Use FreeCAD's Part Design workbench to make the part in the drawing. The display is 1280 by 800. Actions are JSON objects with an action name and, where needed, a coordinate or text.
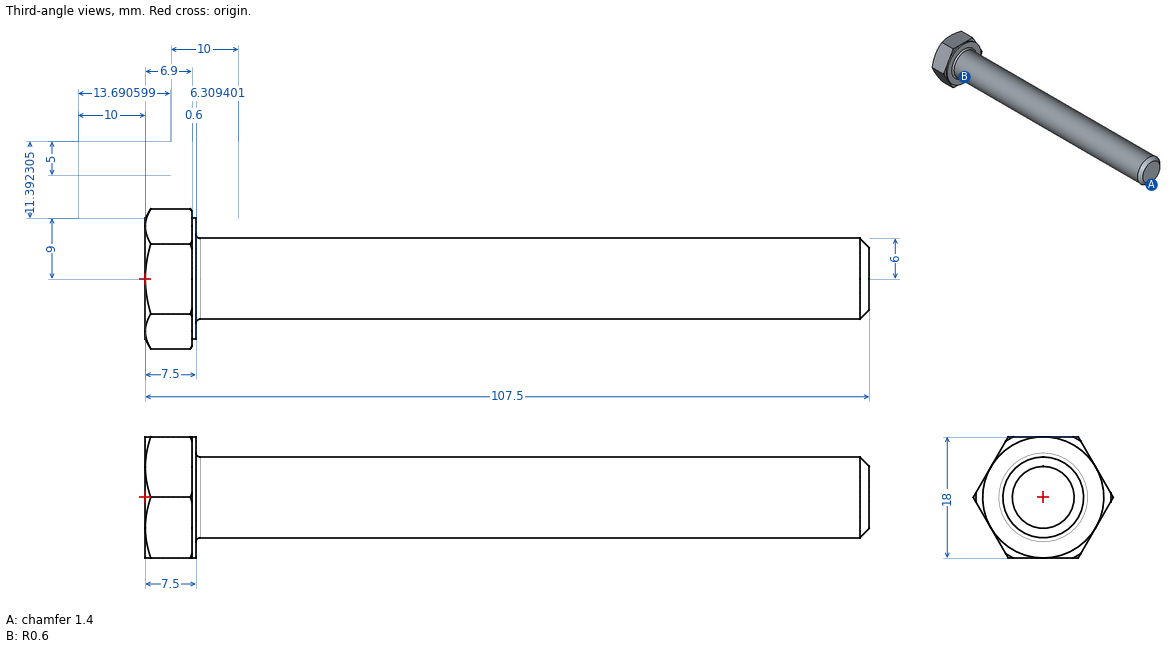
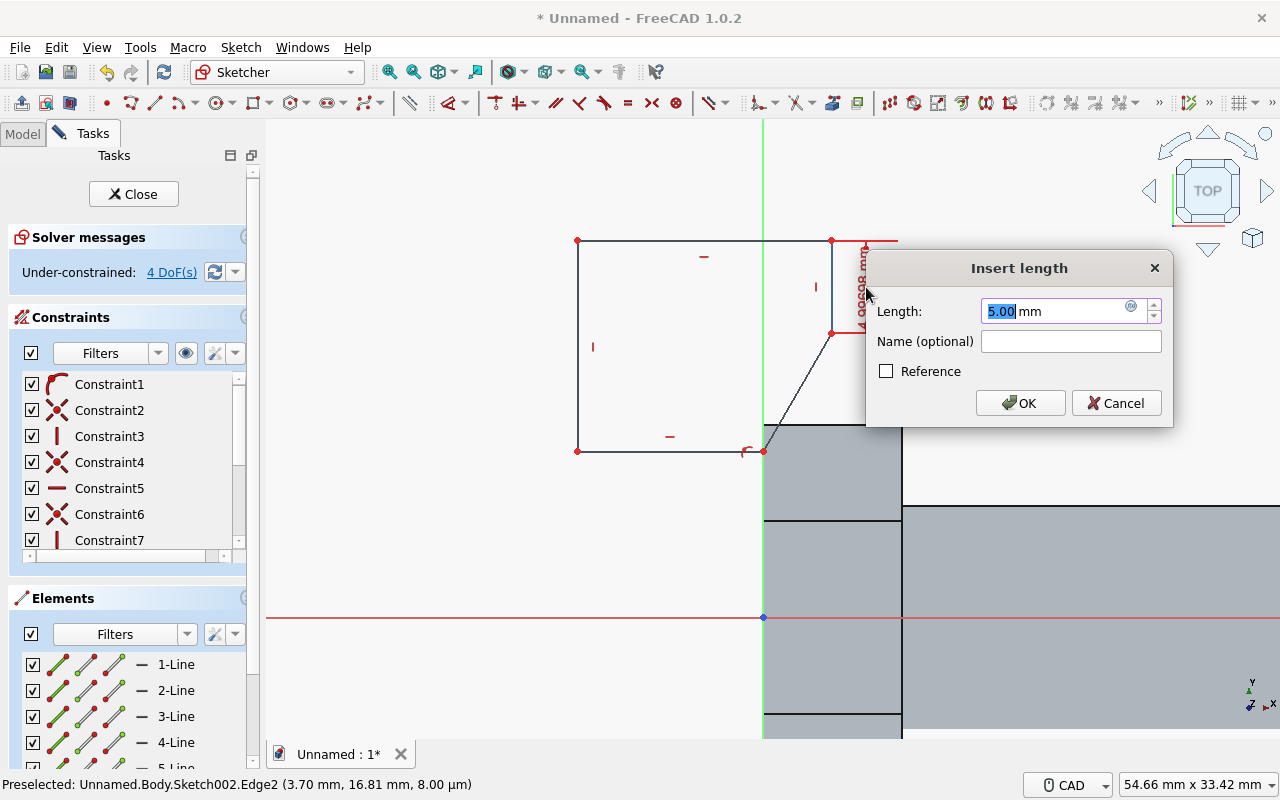
{"action": "type", "text": "5"}
{"action": "key", "text": "Return"}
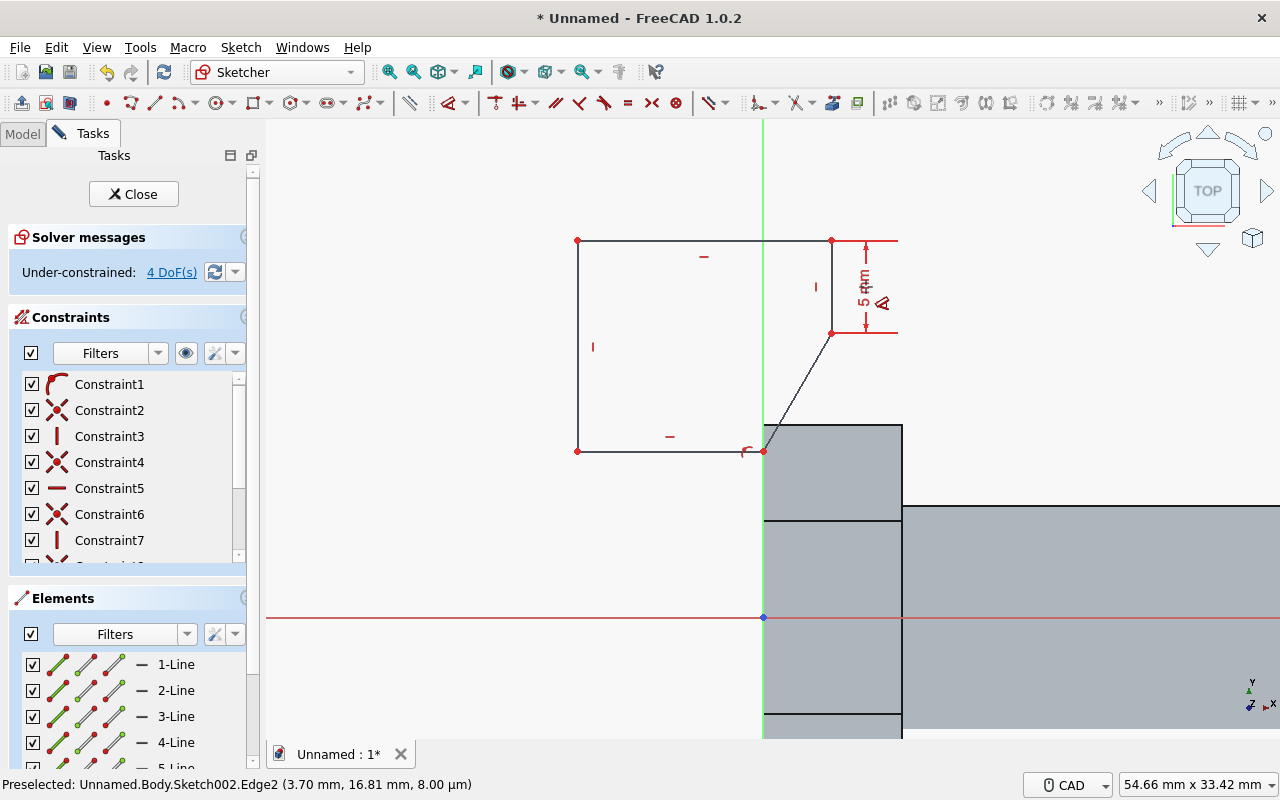
{"action": "left_click", "coordinate": [633, 452]}
{"action": "left_click", "coordinate": [670, 486]}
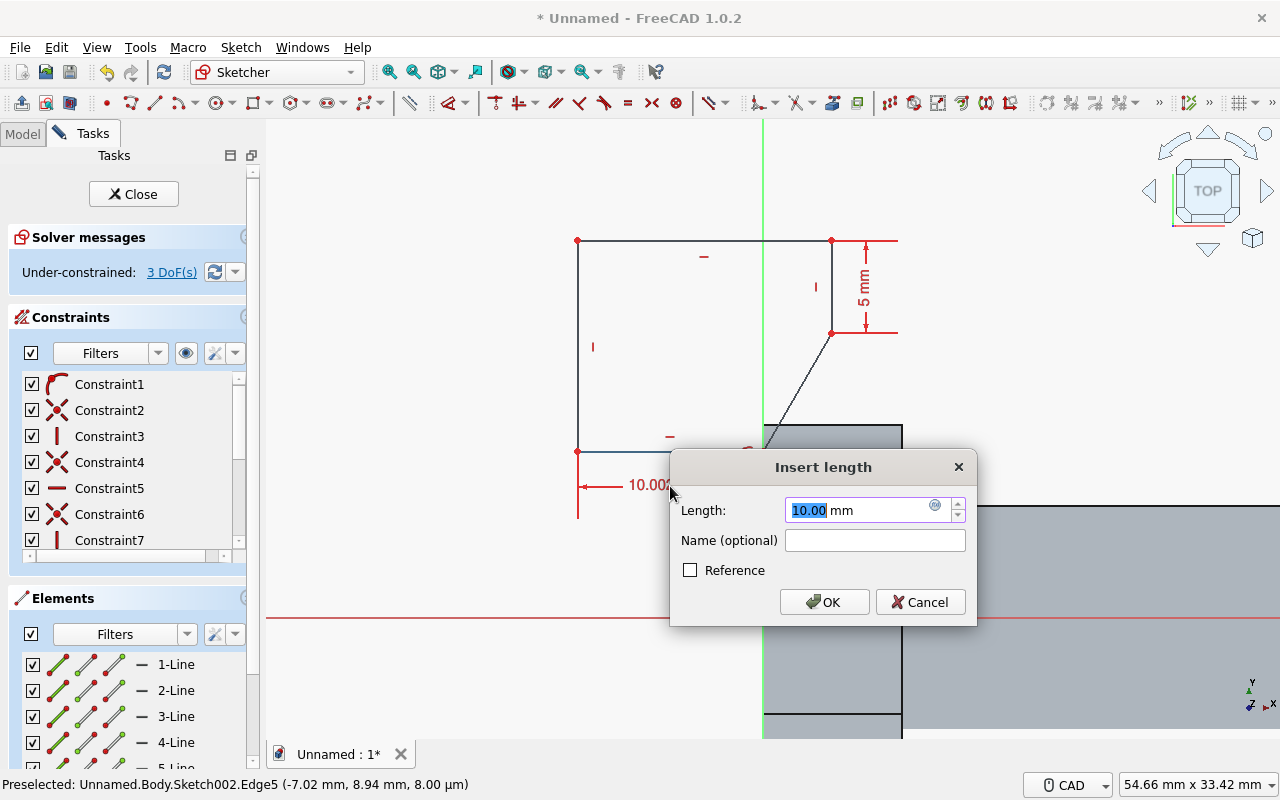
{"action": "type", "text": "10"}
{"action": "key", "text": "Return"}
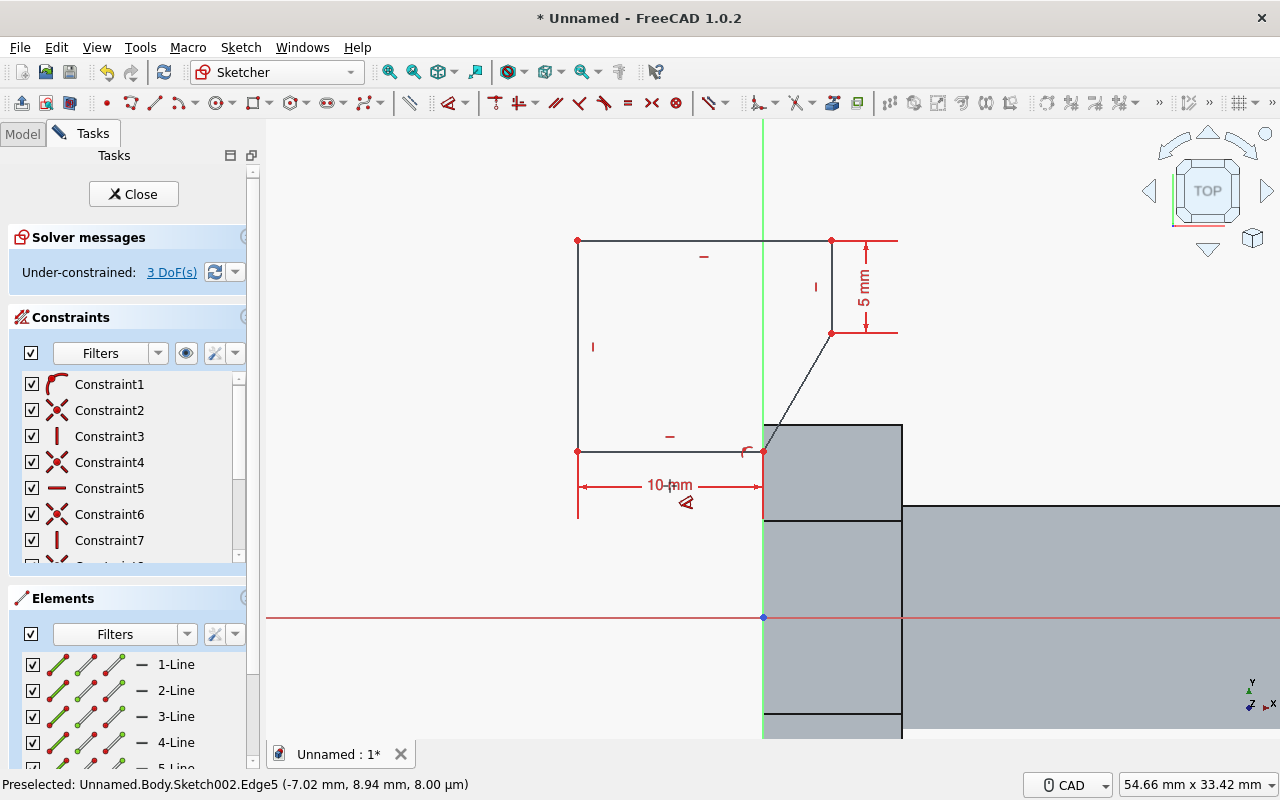
{"action": "left_click", "coordinate": [763, 452]}
{"action": "left_click", "coordinate": [797, 535]}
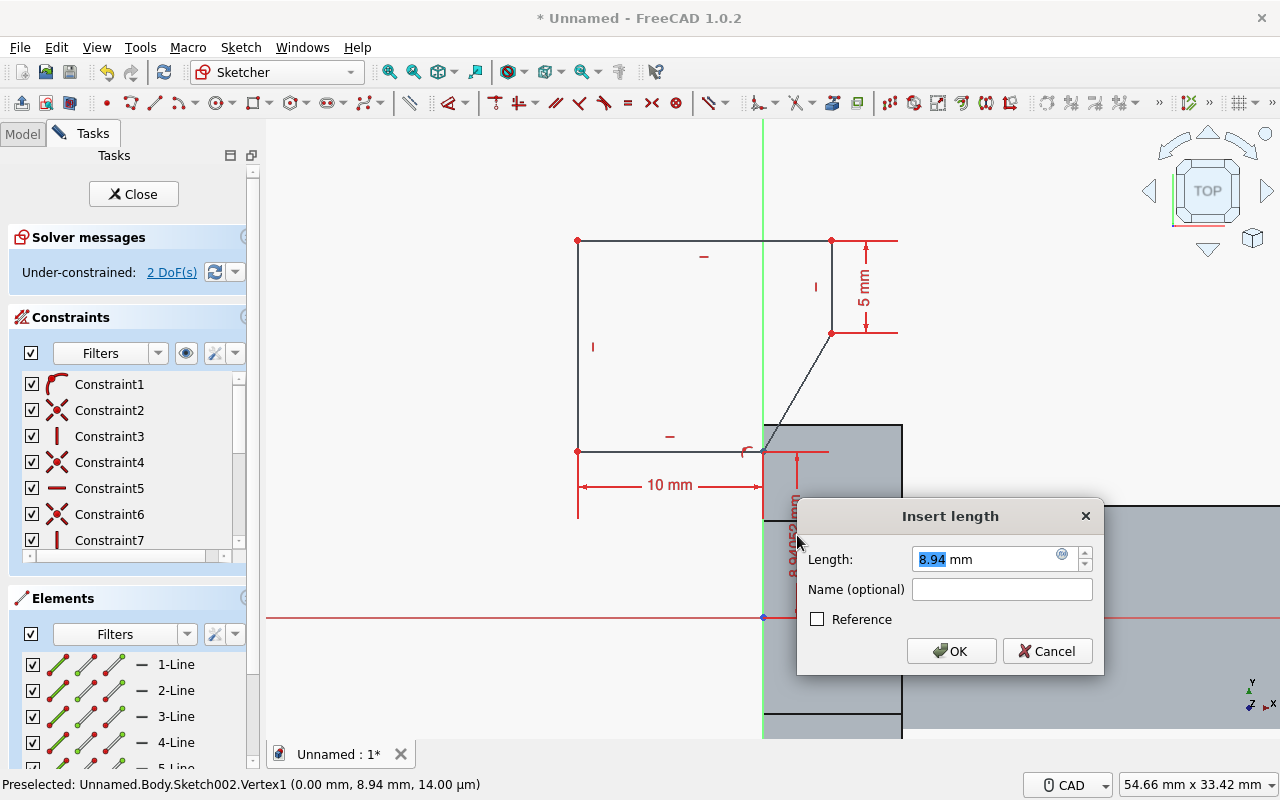
{"action": "type", "text": "9"}
{"action": "key", "text": "Return"}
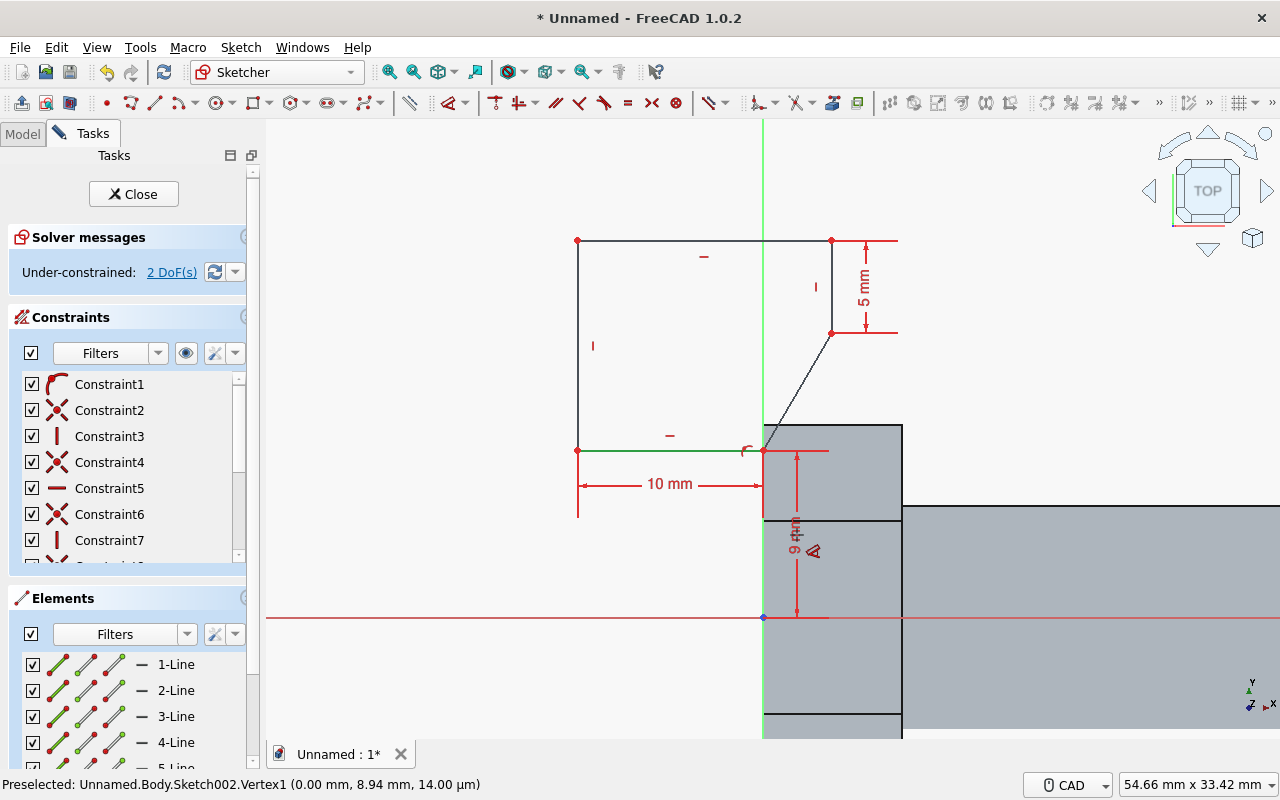
{"action": "left_click", "coordinate": [654, 241]}
{"action": "left_click", "coordinate": [705, 207]}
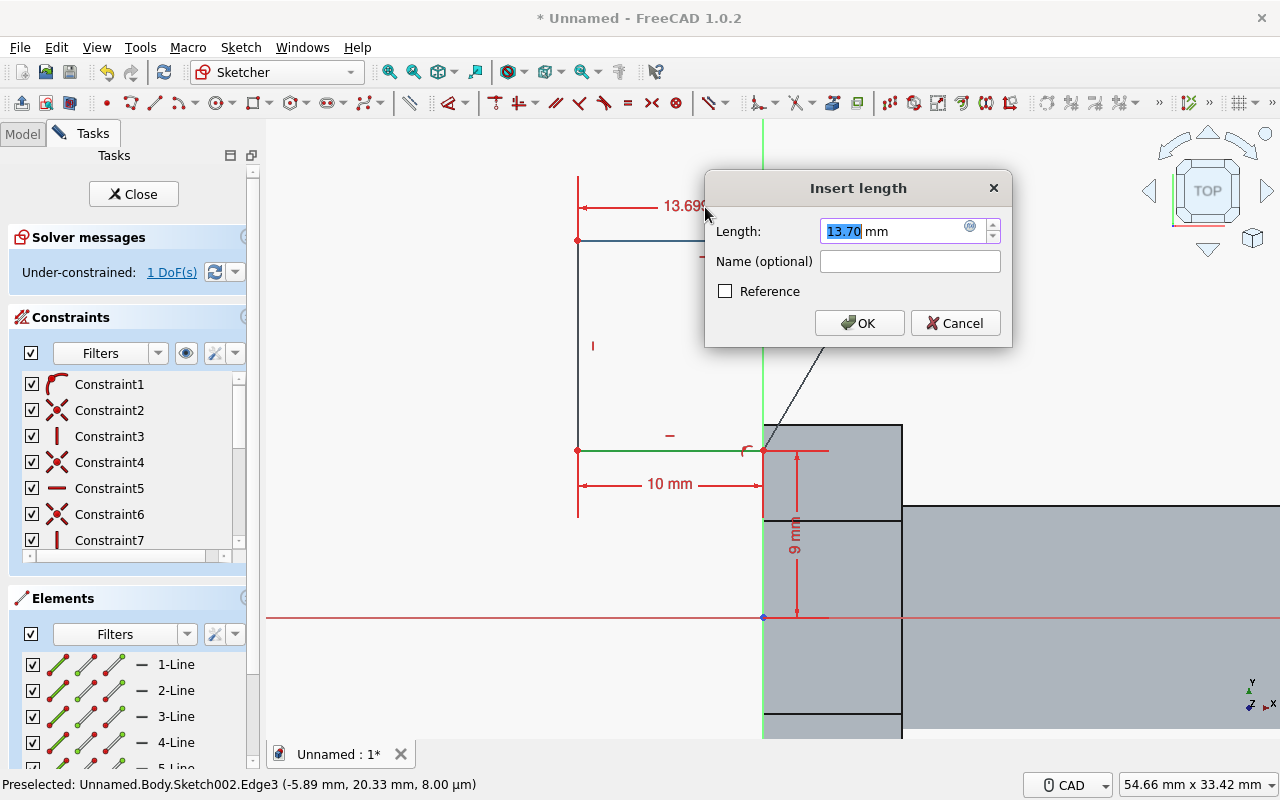
{"action": "type", "text": "13.690599"}
{"action": "key", "text": "Return"}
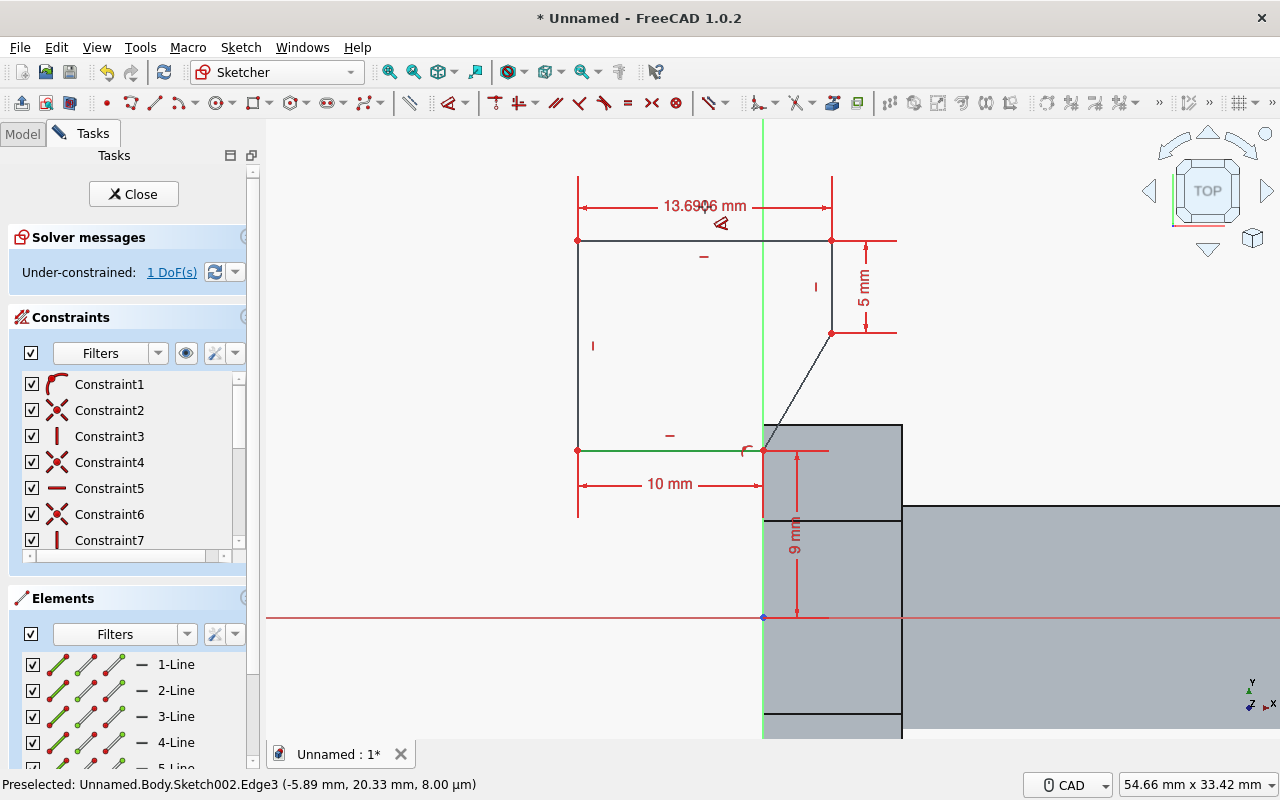
{"action": "left_click", "coordinate": [578, 304]}
{"action": "left_click", "coordinate": [544, 346]}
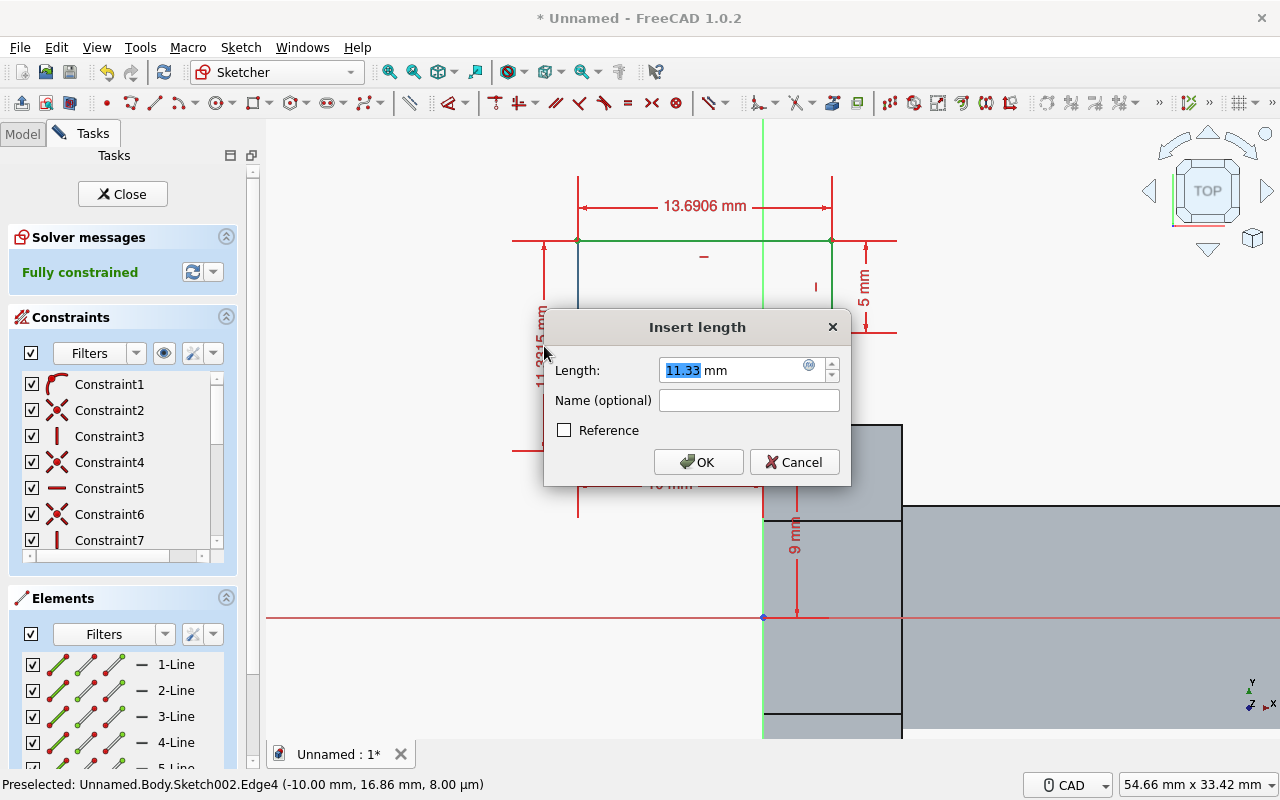
{"action": "type", "text": "11.392305"}
{"action": "key", "text": "Return"}
{"action": "key", "text": "Escape"}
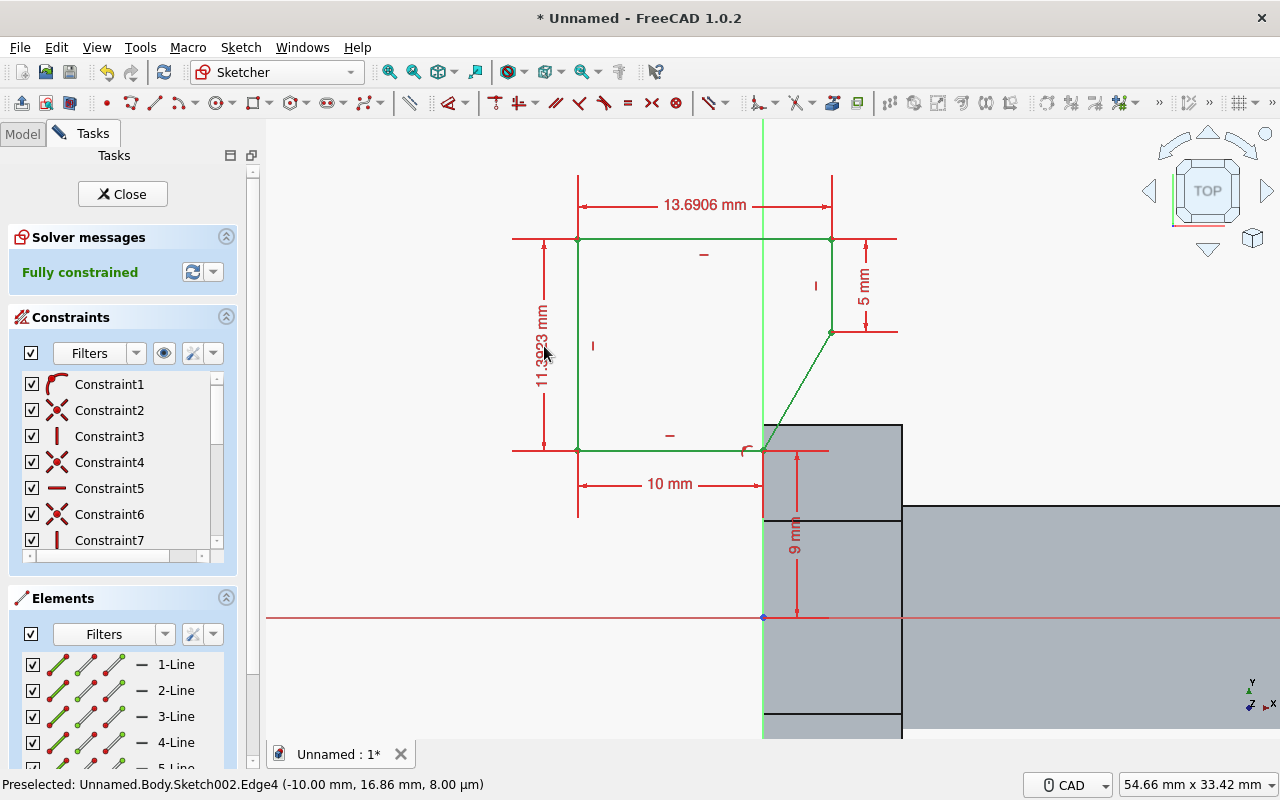
{"action": "left_click", "coordinate": [123, 194]}